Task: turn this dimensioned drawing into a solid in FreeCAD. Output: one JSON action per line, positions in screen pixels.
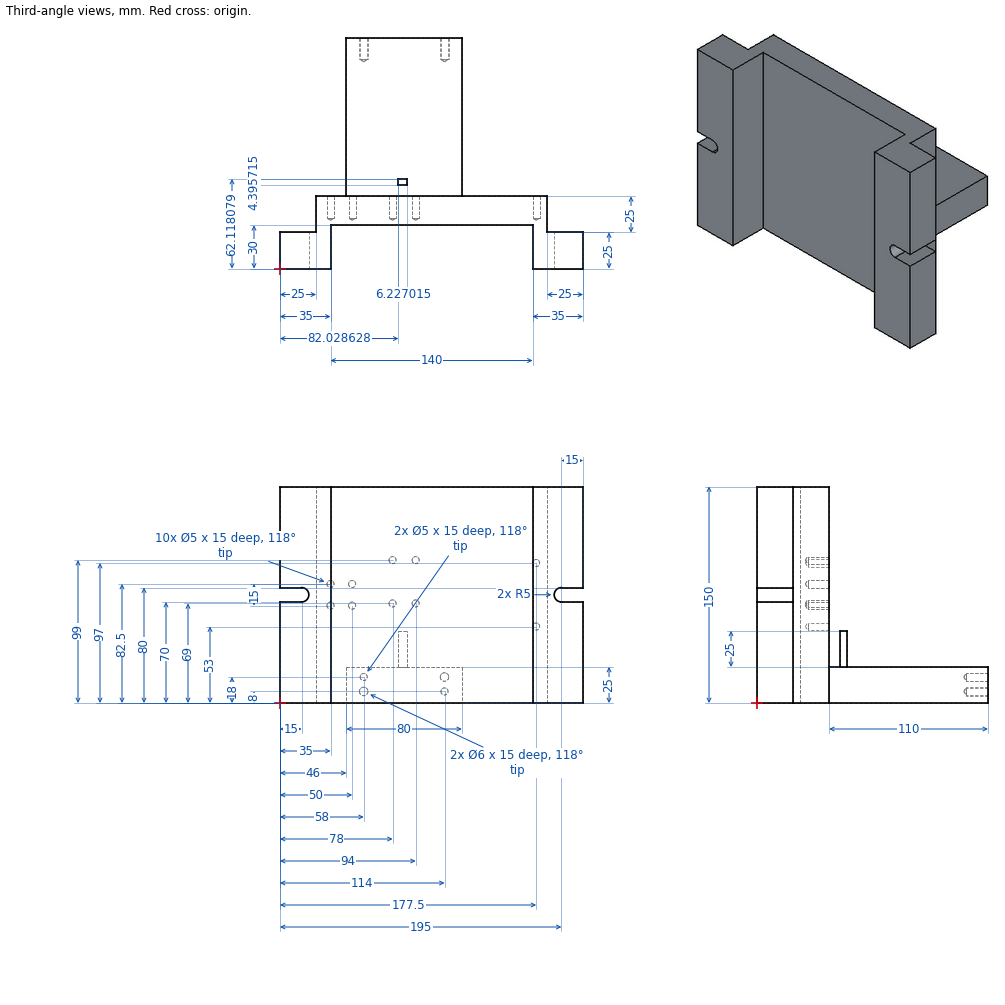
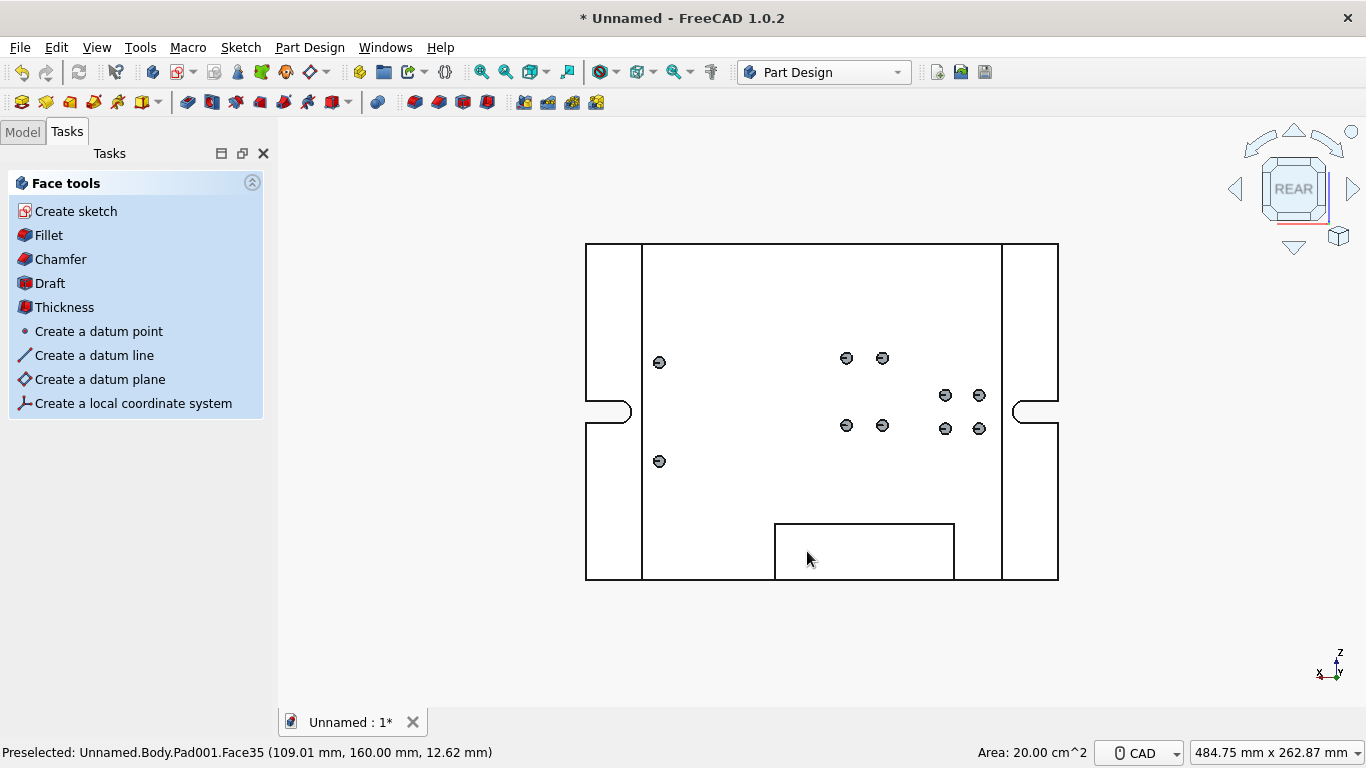
{"action": "left_click", "coordinate": [178, 72]}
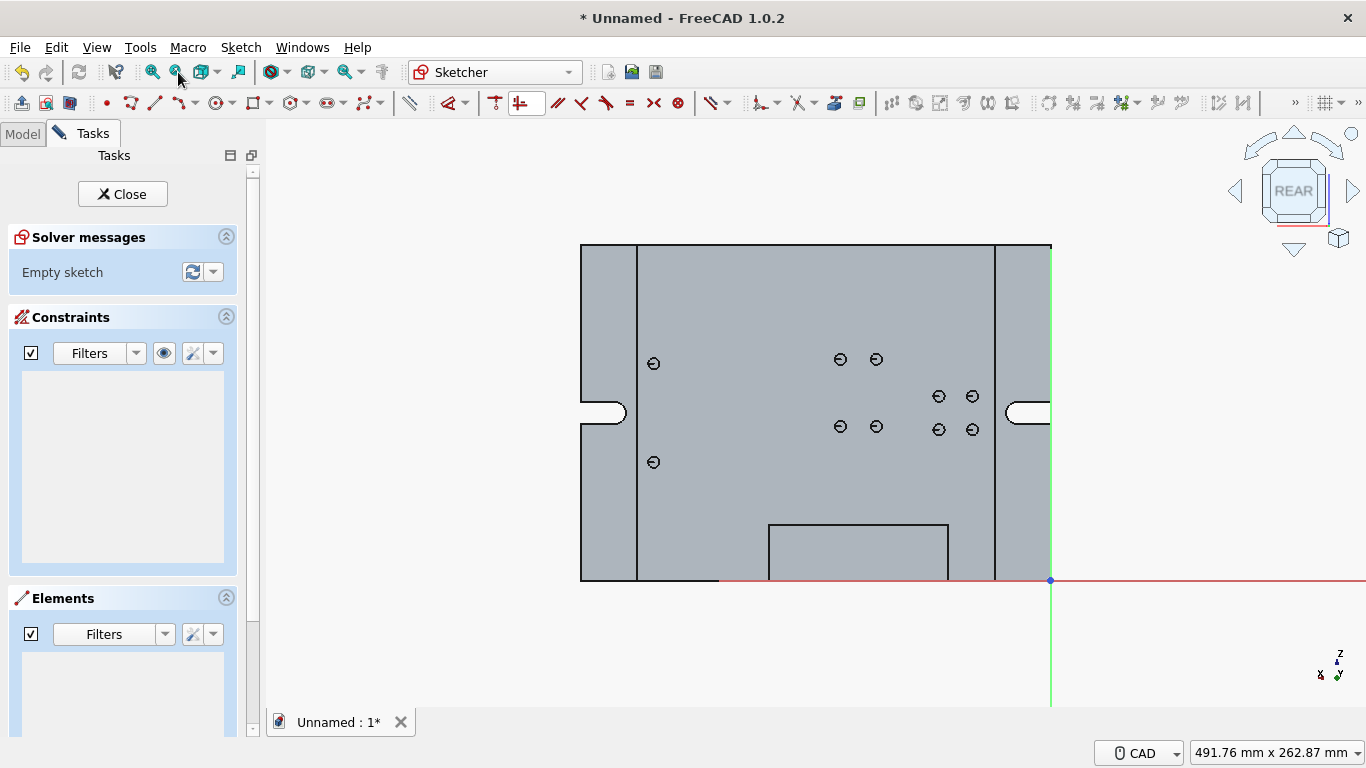
{"action": "scroll", "coordinate": [1062, 676], "scroll_direction": "up", "scroll_amount": 4}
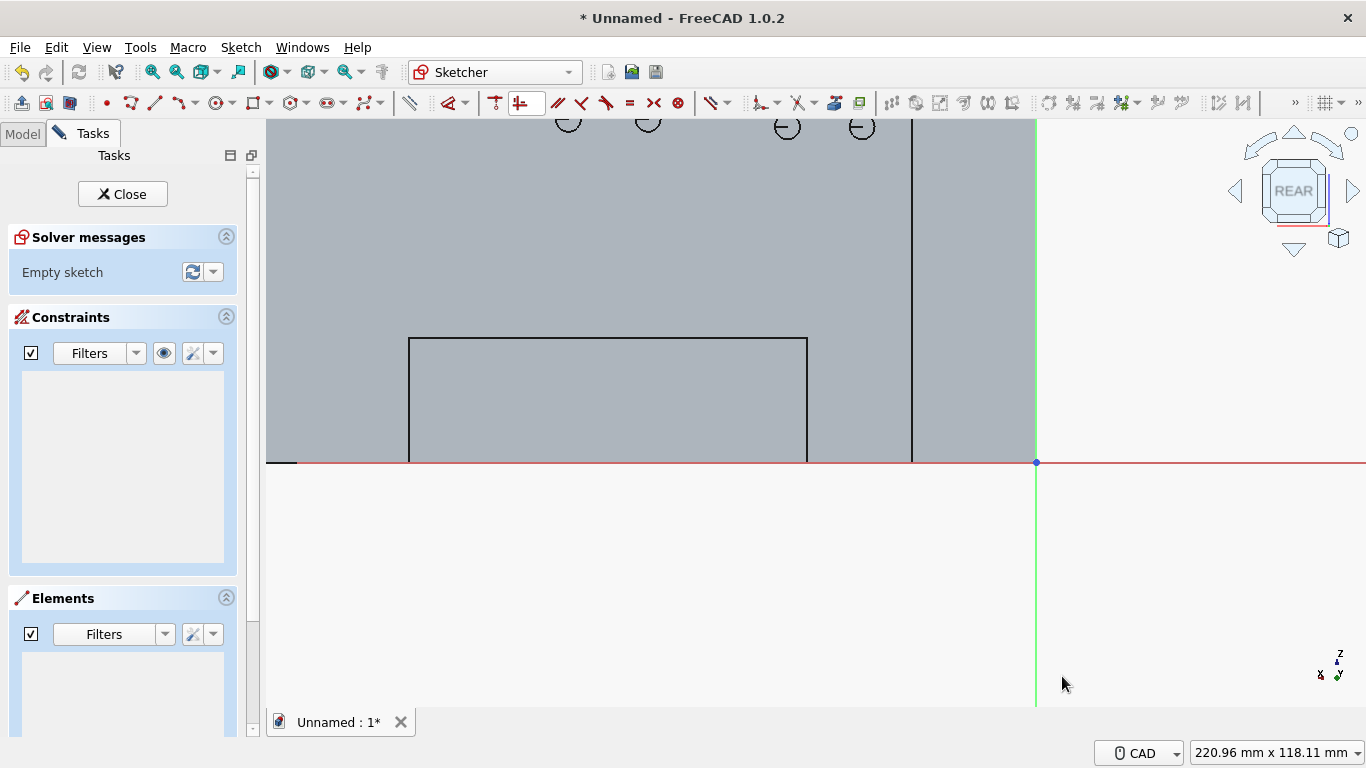
{"action": "key", "text": "g c"}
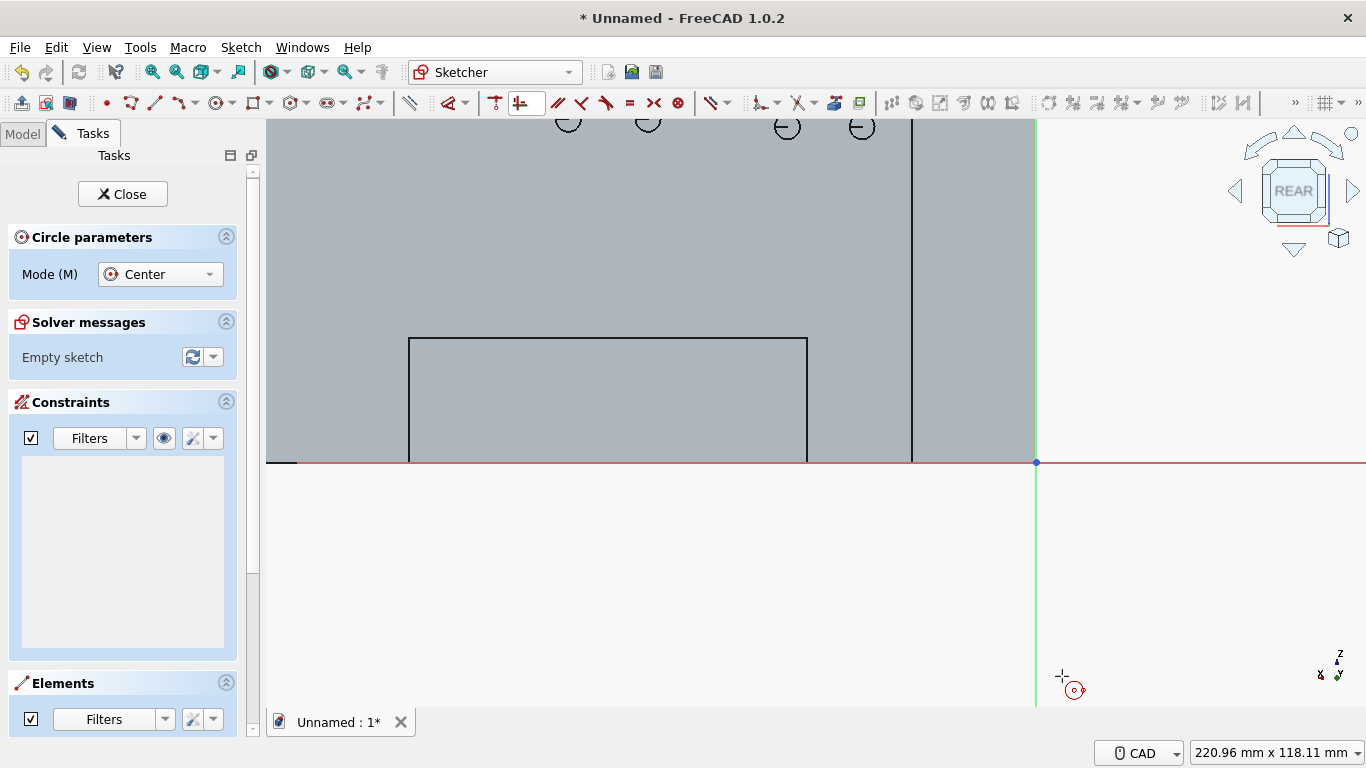
{"action": "scroll", "coordinate": [748, 373], "scroll_direction": "up", "scroll_amount": 4}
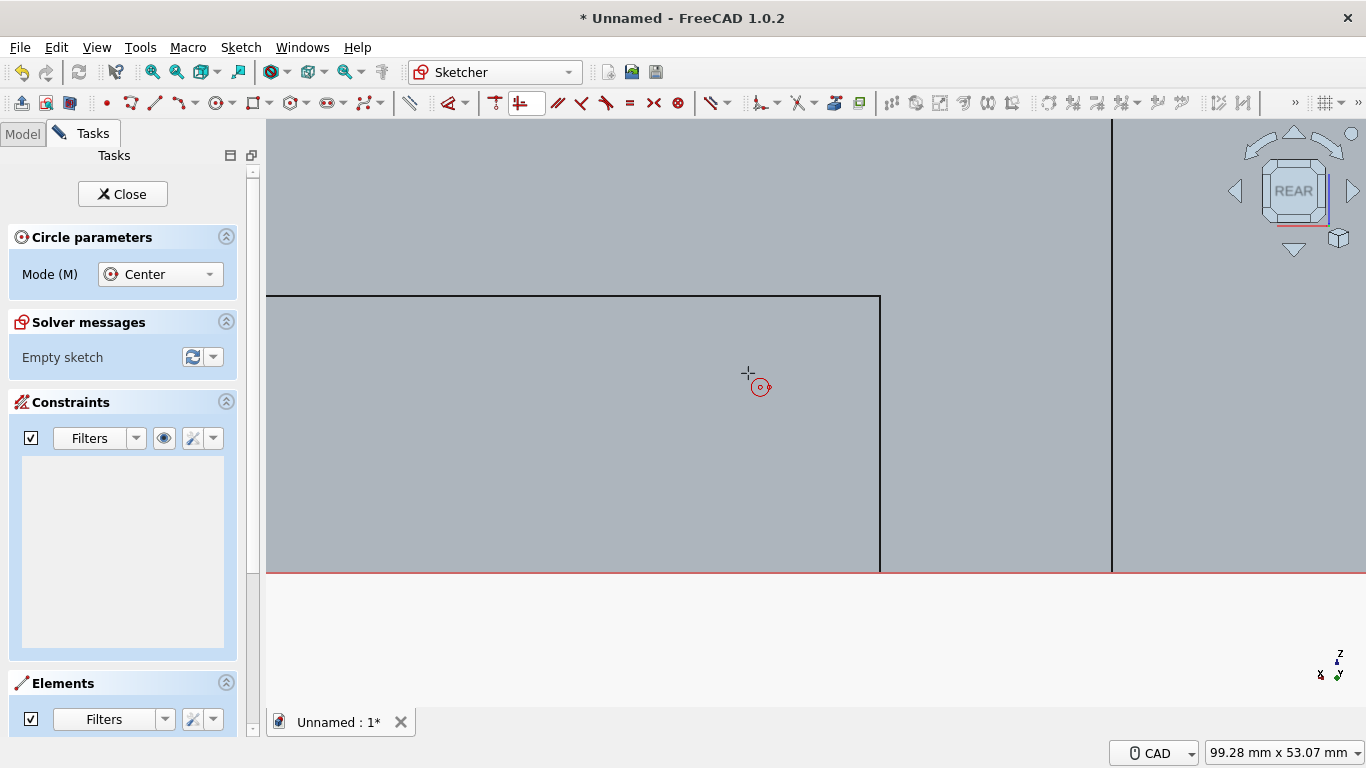
{"action": "left_click", "coordinate": [747, 373]}
{"action": "mouse_move", "coordinate": [766, 354]}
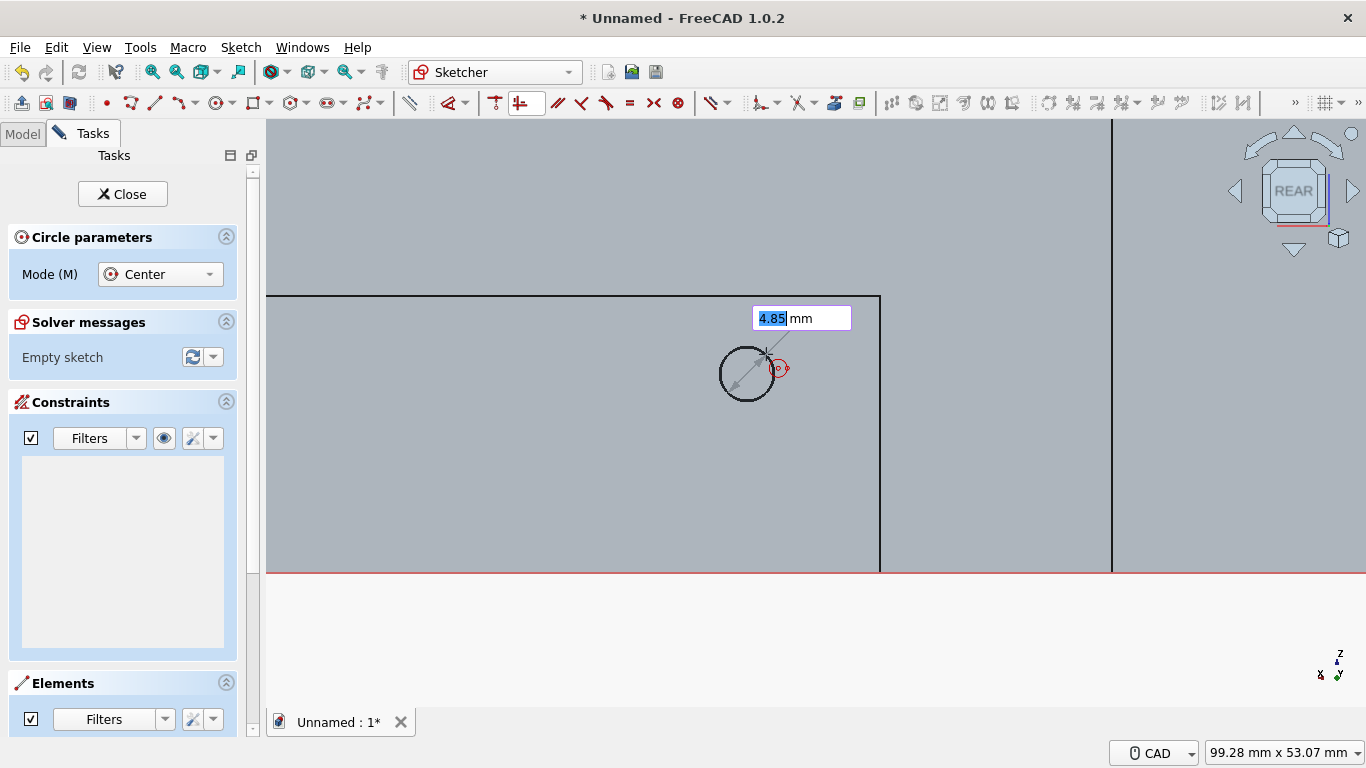
{"action": "type", "text": "5"}
{"action": "key", "text": "Return"}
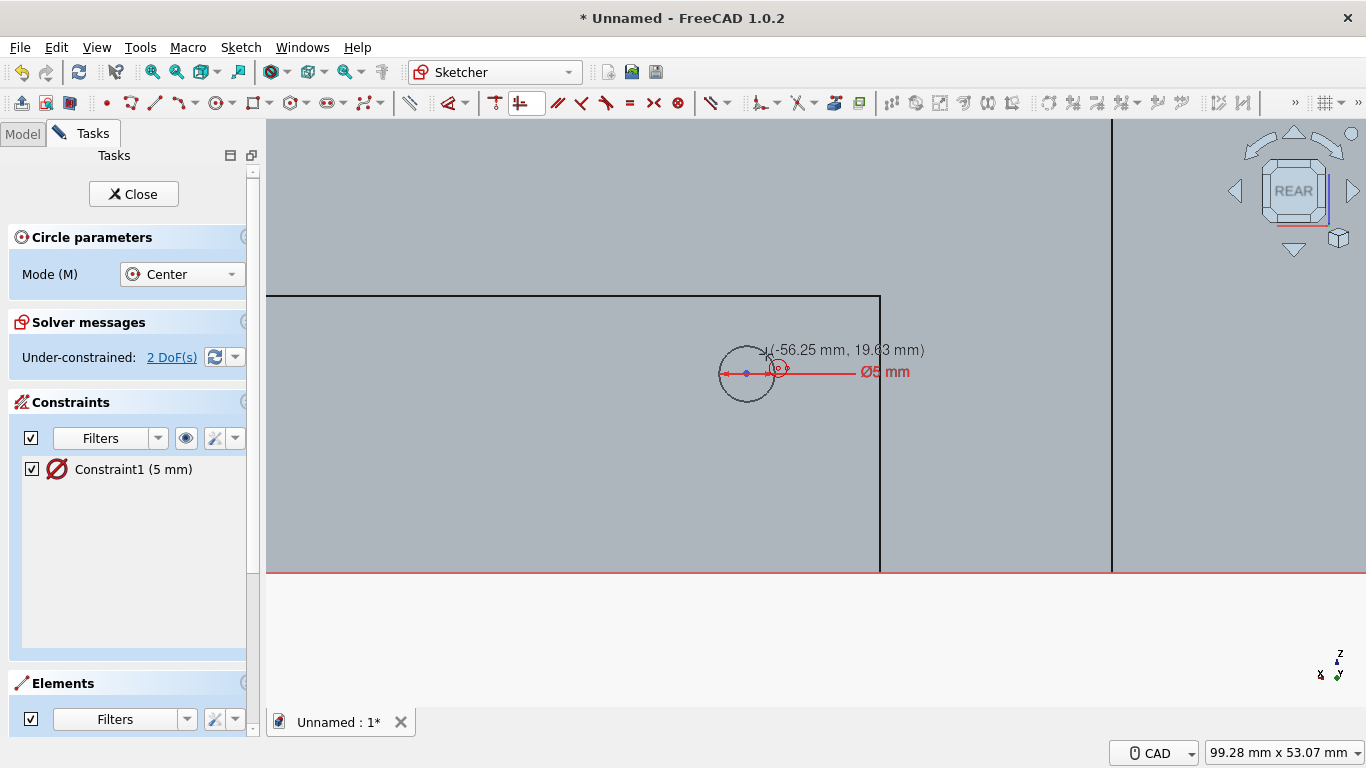
{"action": "scroll", "coordinate": [751, 376], "scroll_direction": "down", "scroll_amount": 4}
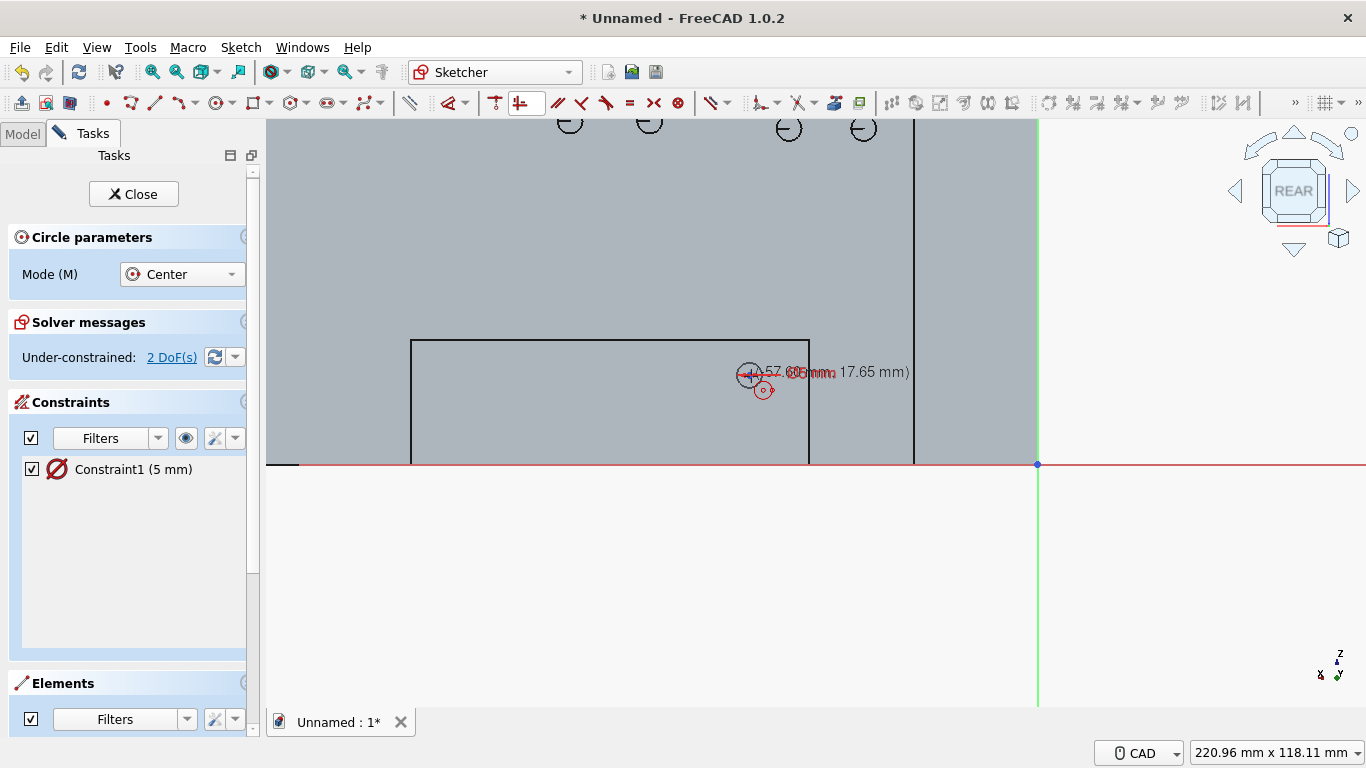
{"action": "scroll", "coordinate": [470, 425], "scroll_direction": "up", "scroll_amount": 4}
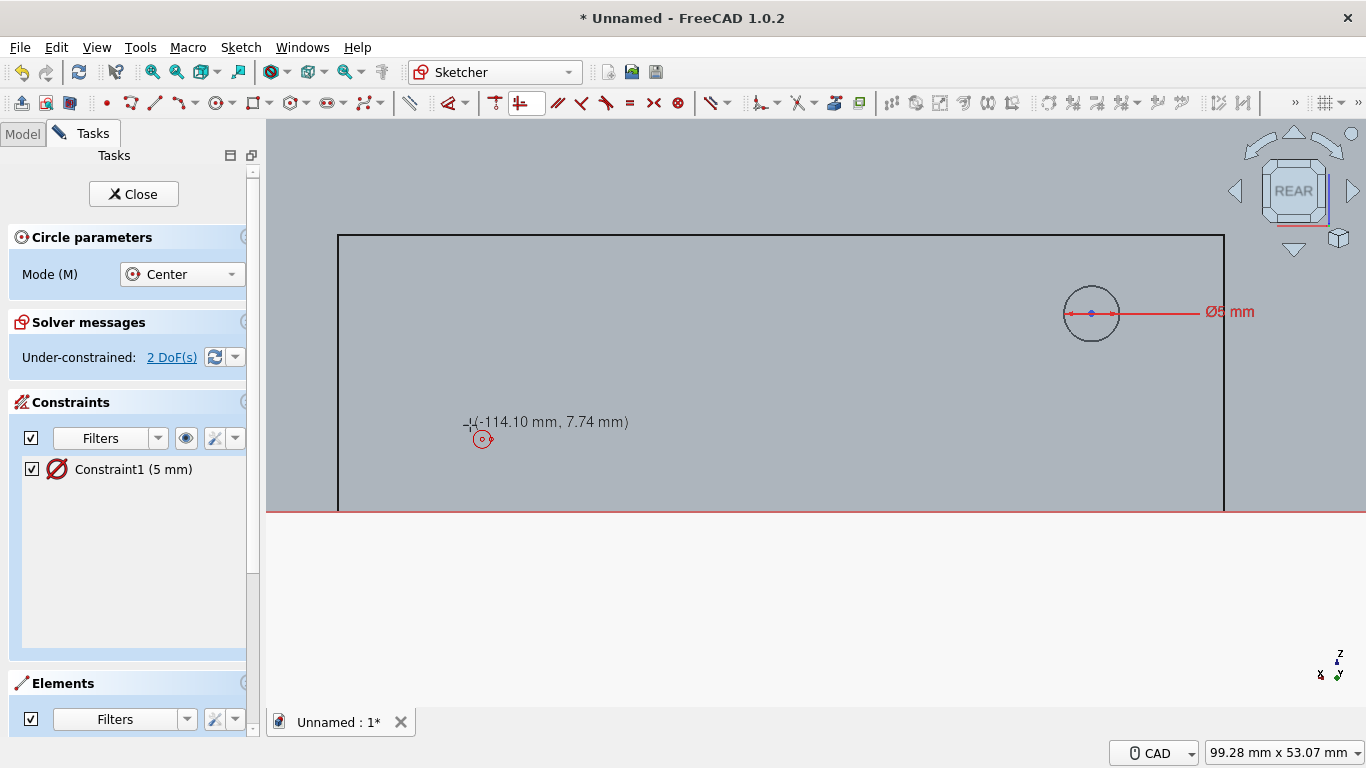
{"action": "left_click", "coordinate": [471, 424]}
{"action": "mouse_move", "coordinate": [490, 404]}